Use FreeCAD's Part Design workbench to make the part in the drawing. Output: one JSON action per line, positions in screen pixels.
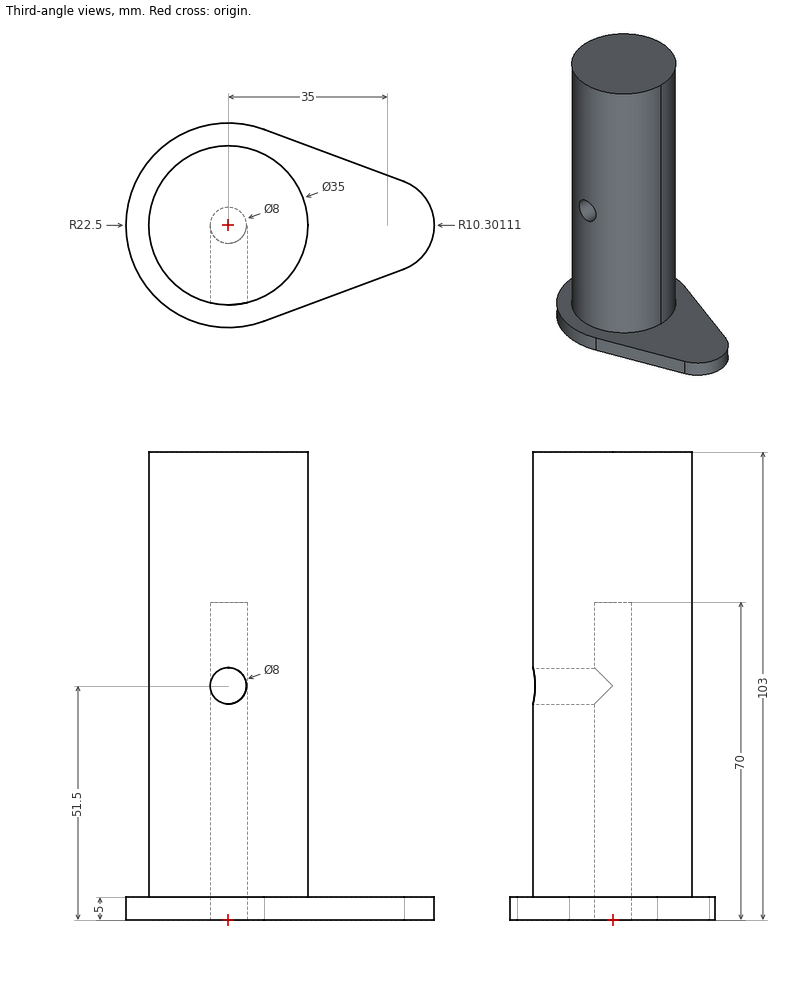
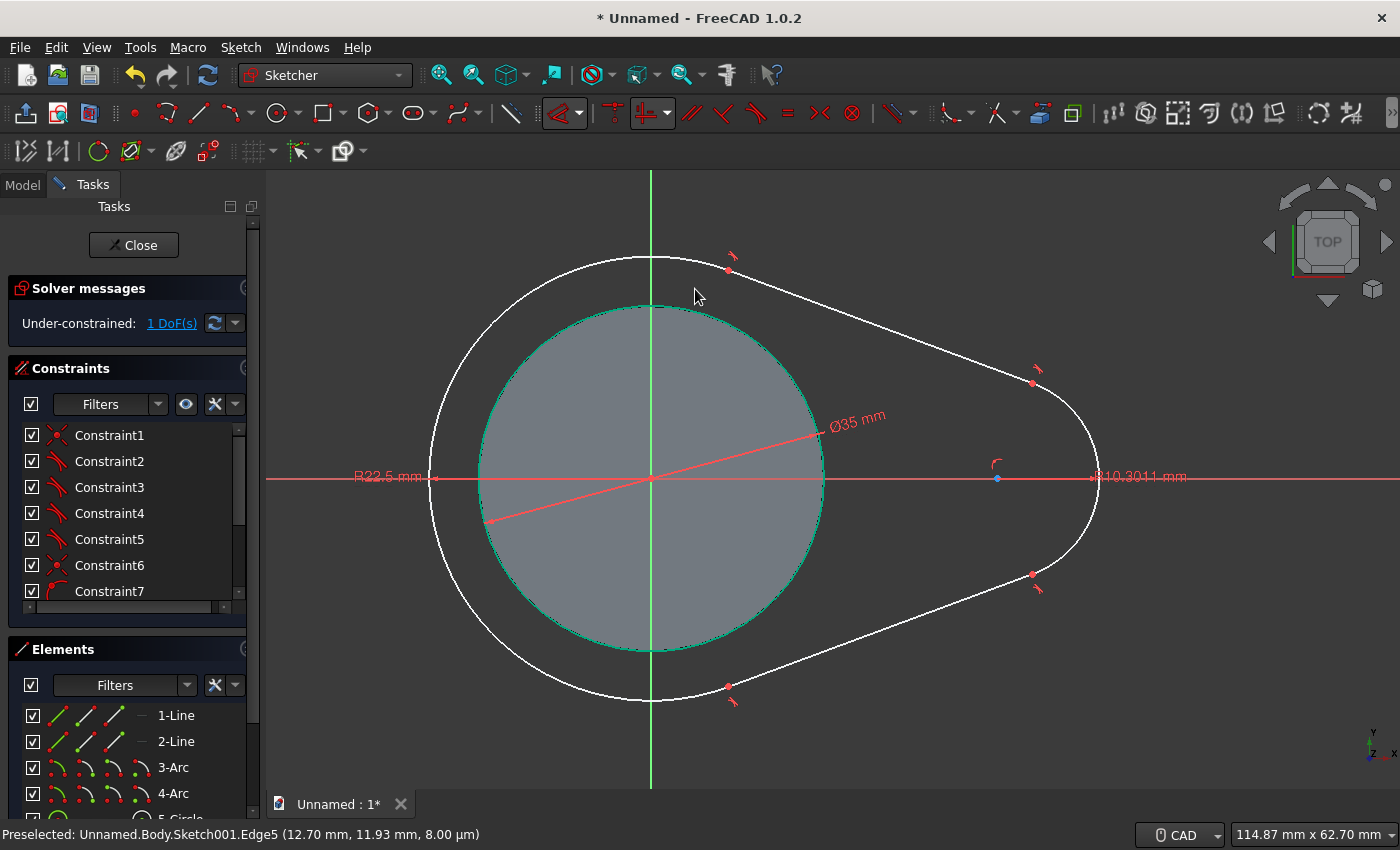
{"action": "left_click", "coordinate": [997, 479]}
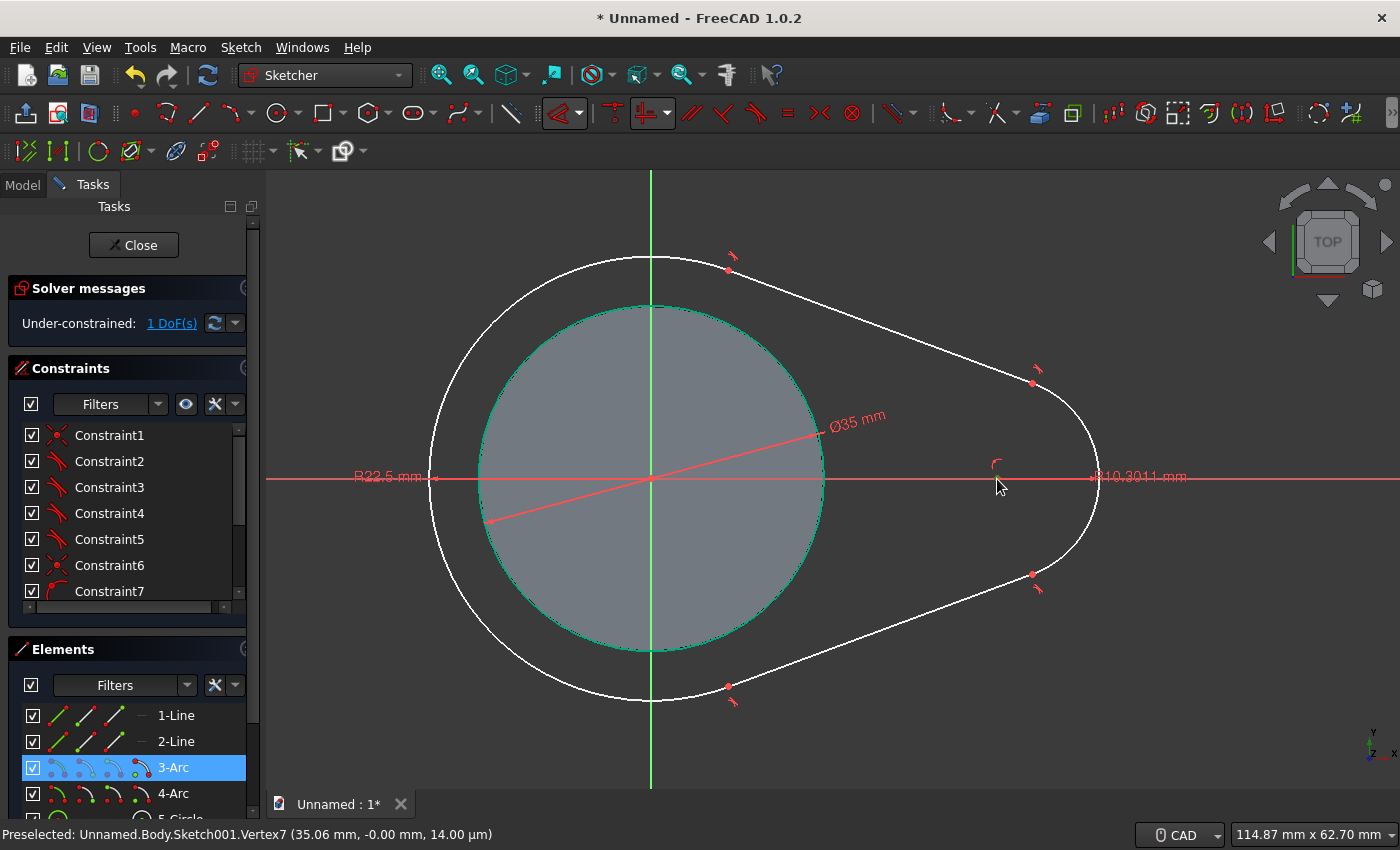
{"action": "key", "text": "l"}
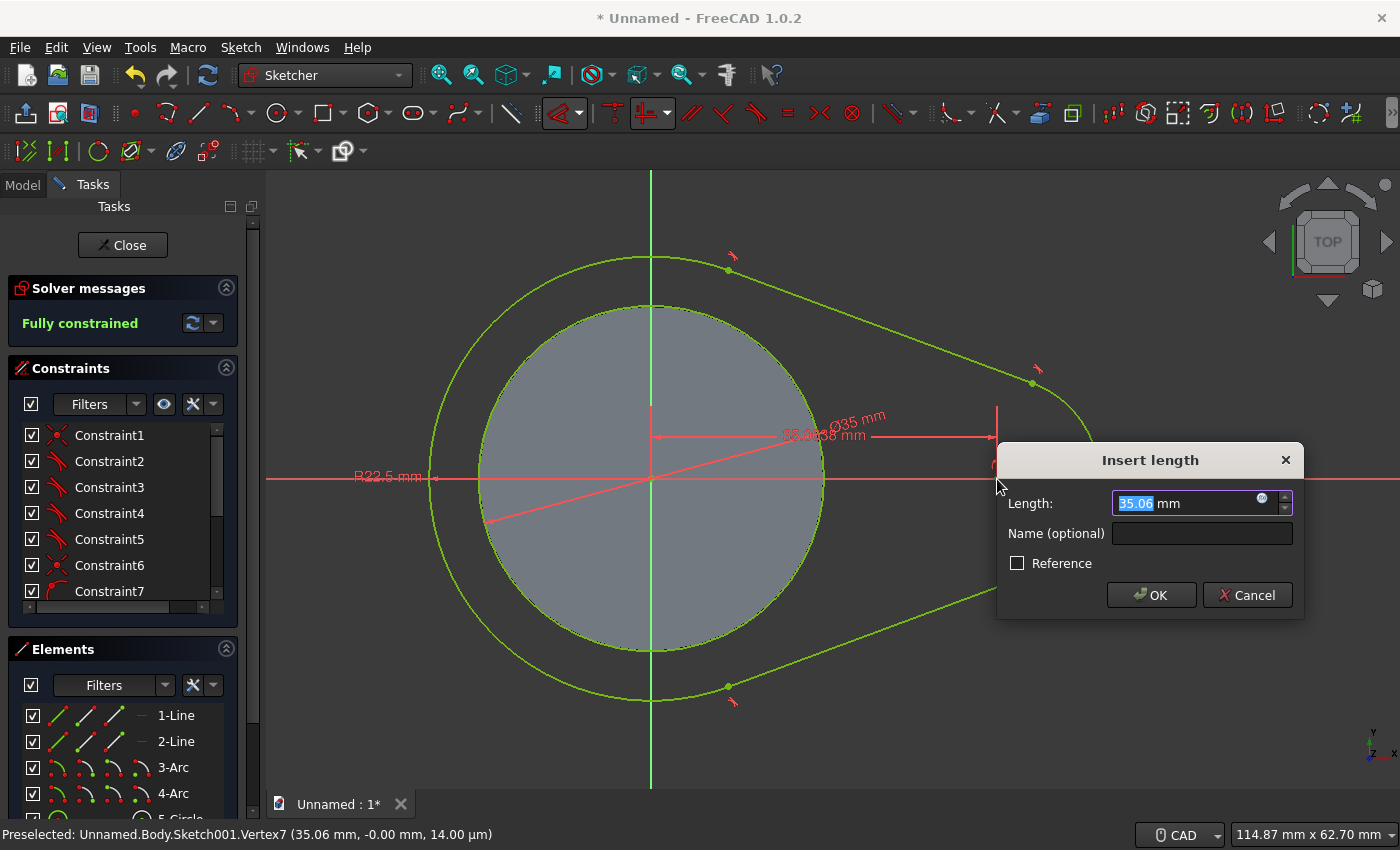
{"action": "type", "text": "35"}
{"action": "key", "text": "Return"}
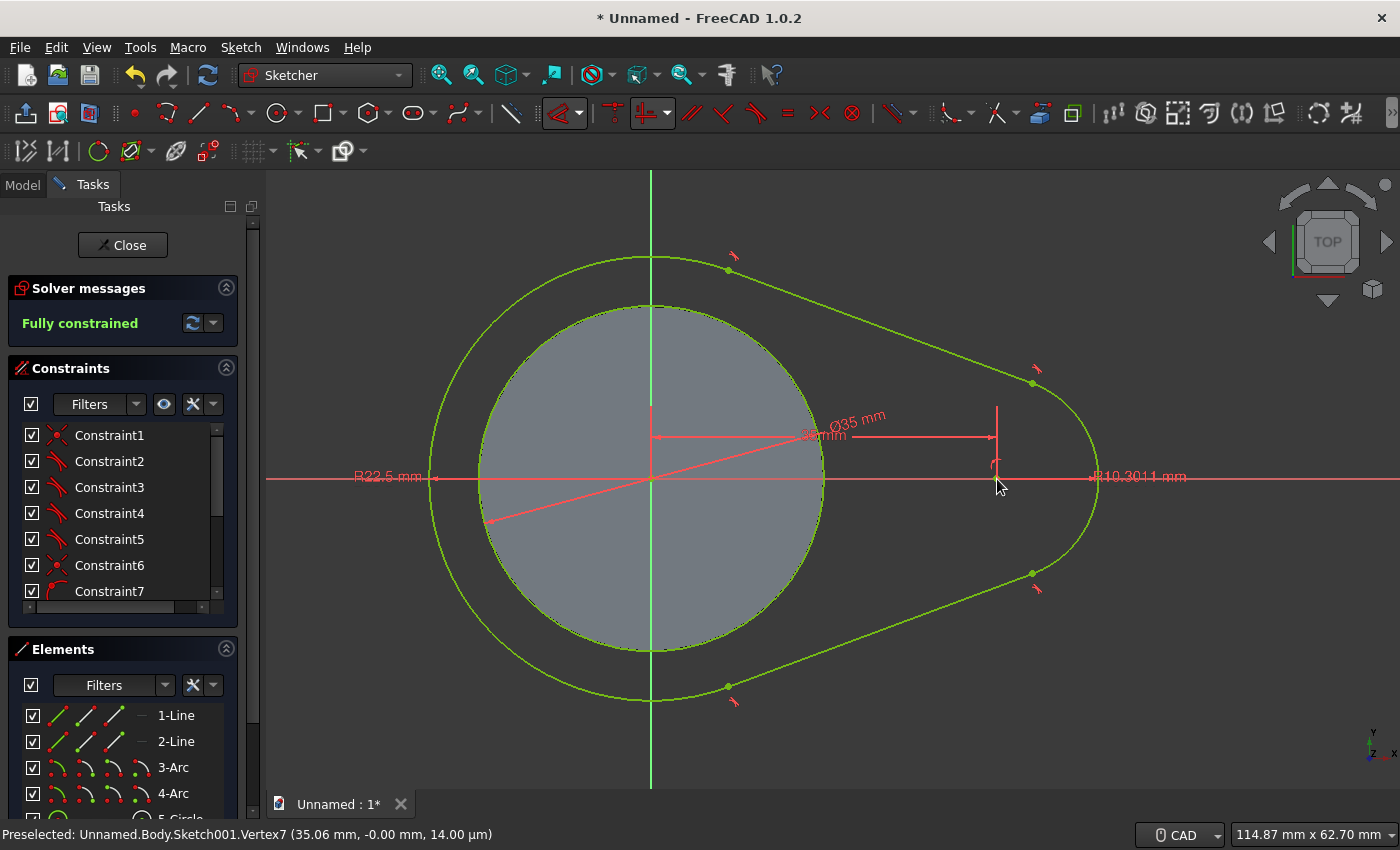
{"action": "left_click", "coordinate": [123, 245]}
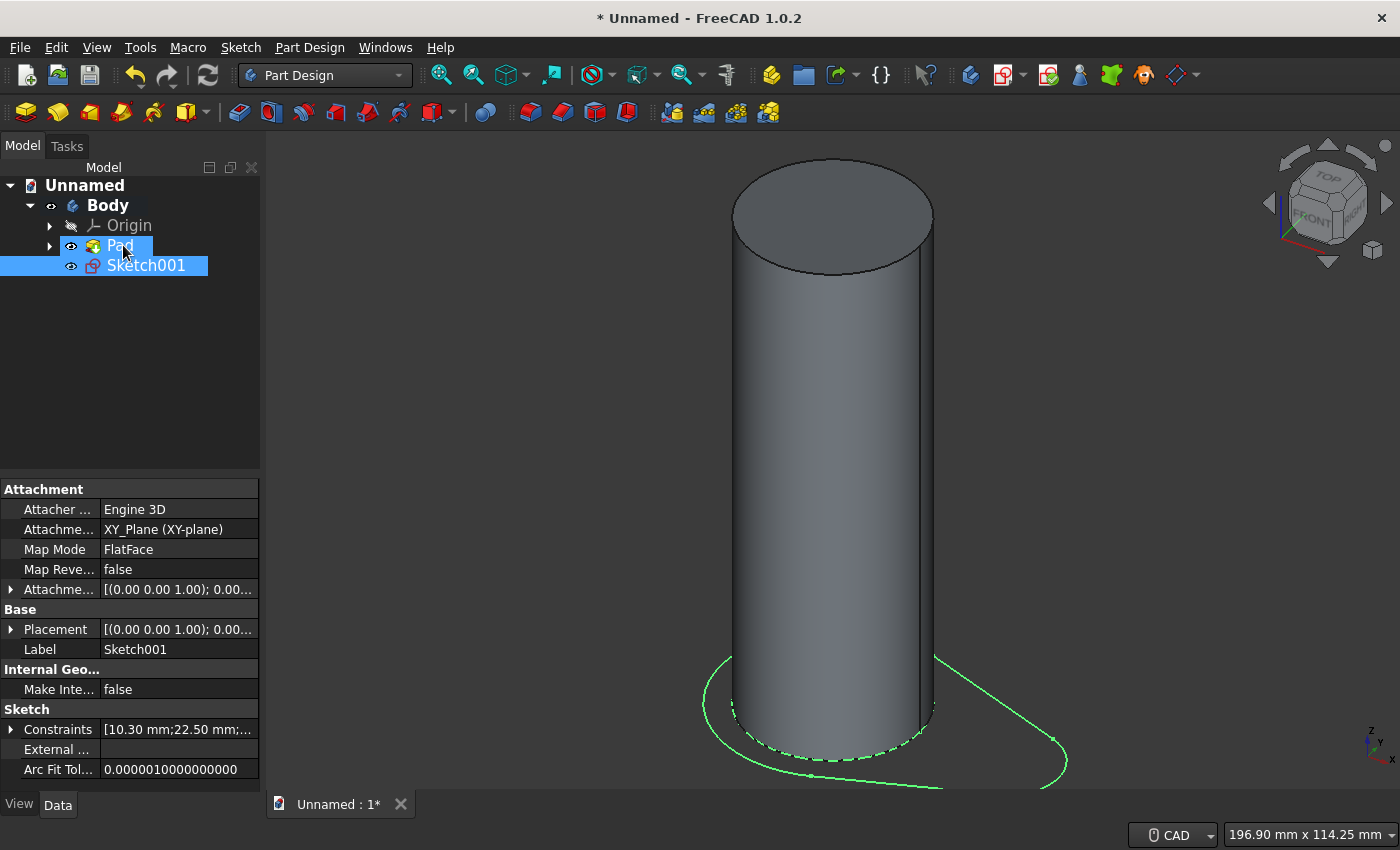
{"action": "left_click", "coordinate": [26, 112]}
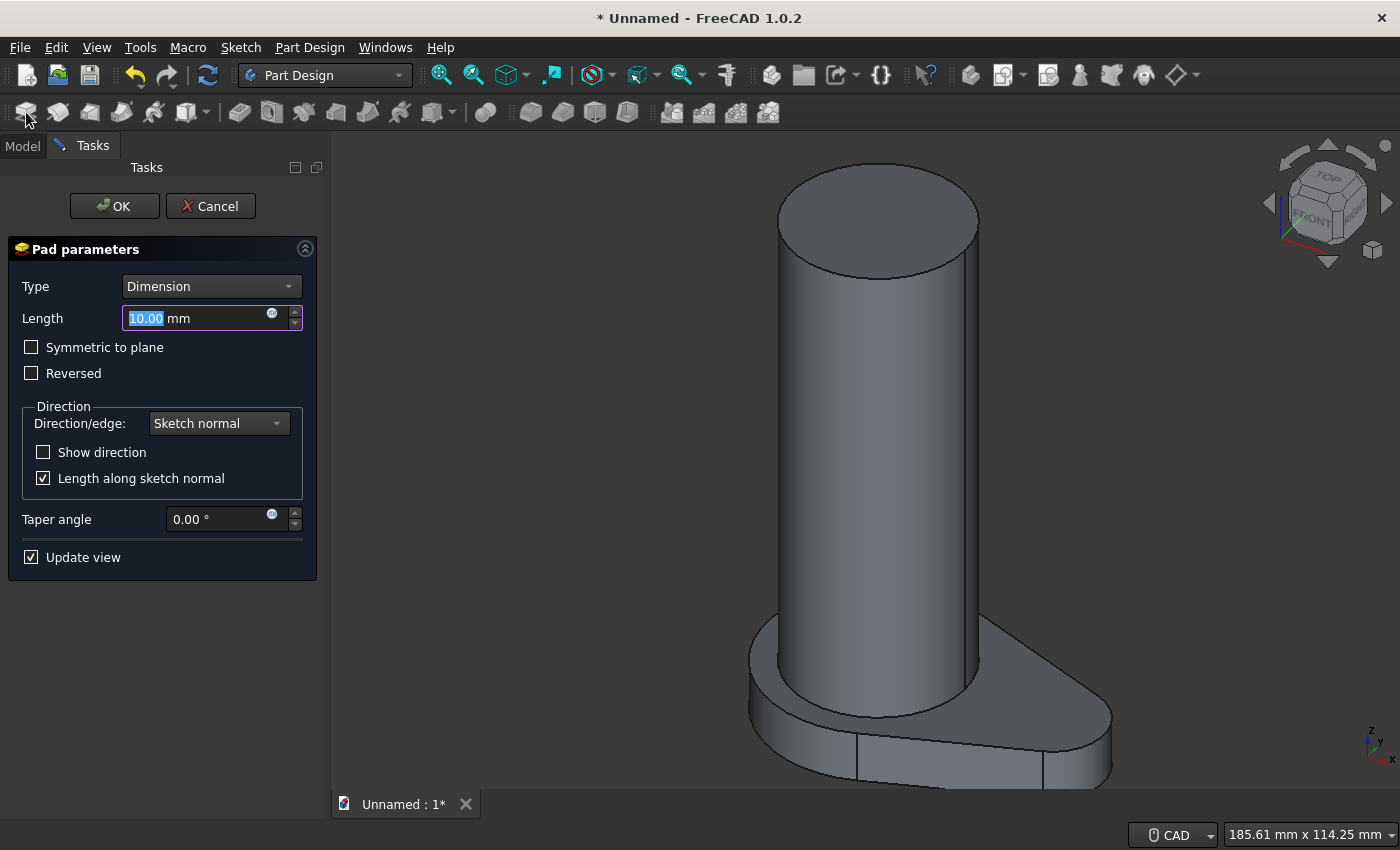
{"action": "type", "text": "5"}
{"action": "key", "text": "Tab"}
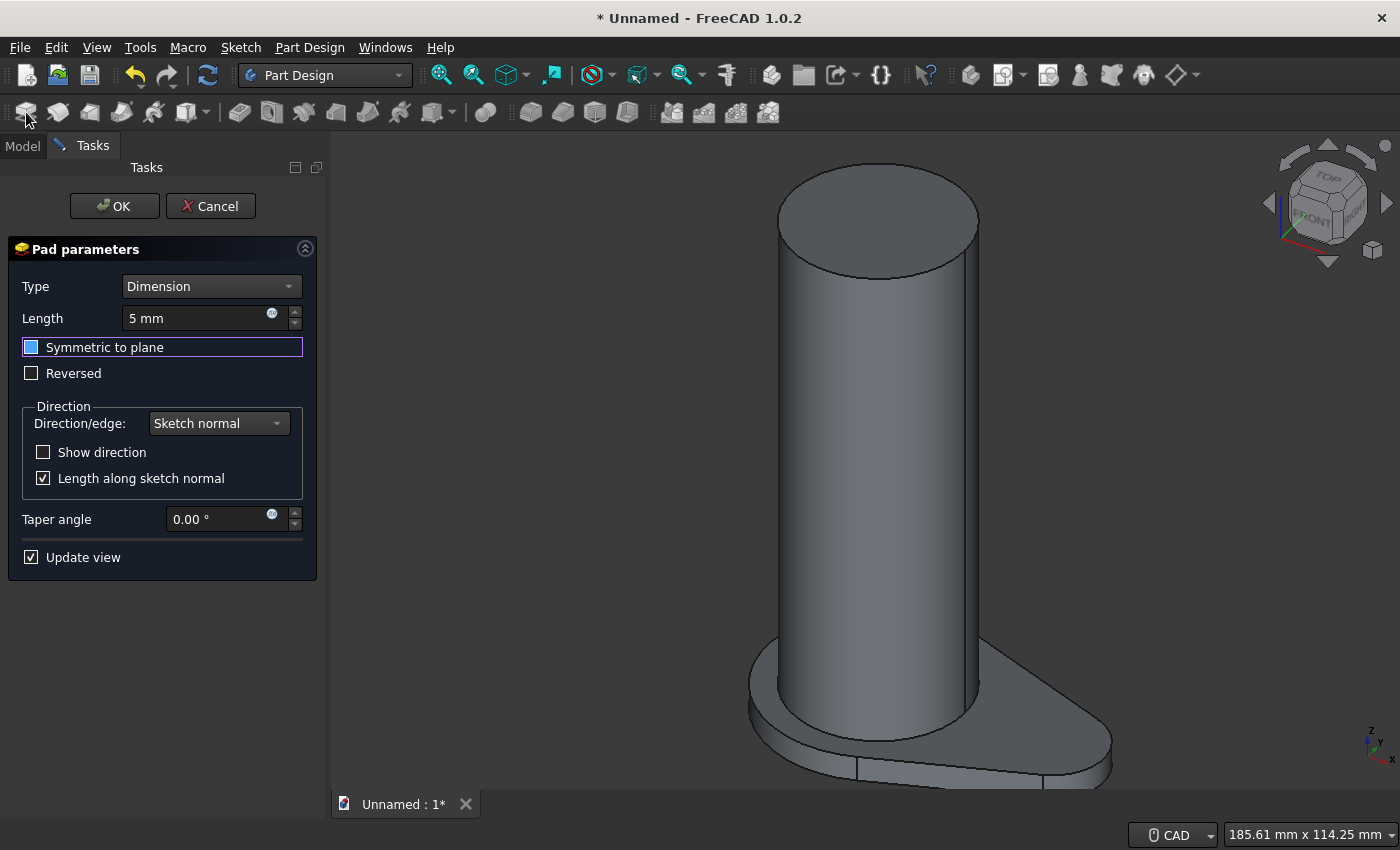
{"action": "left_click", "coordinate": [115, 206]}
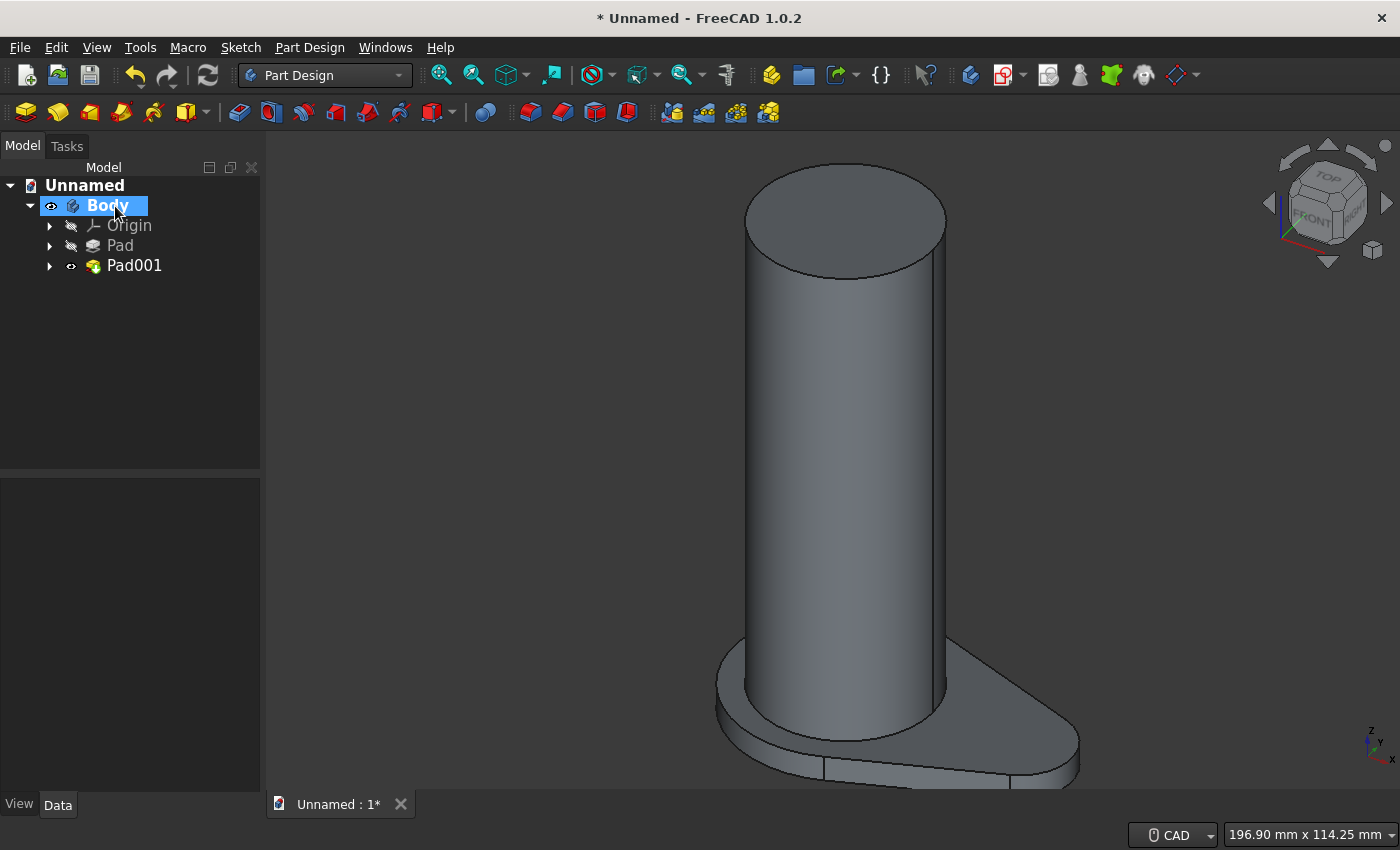
{"action": "left_click", "coordinate": [442, 76]}